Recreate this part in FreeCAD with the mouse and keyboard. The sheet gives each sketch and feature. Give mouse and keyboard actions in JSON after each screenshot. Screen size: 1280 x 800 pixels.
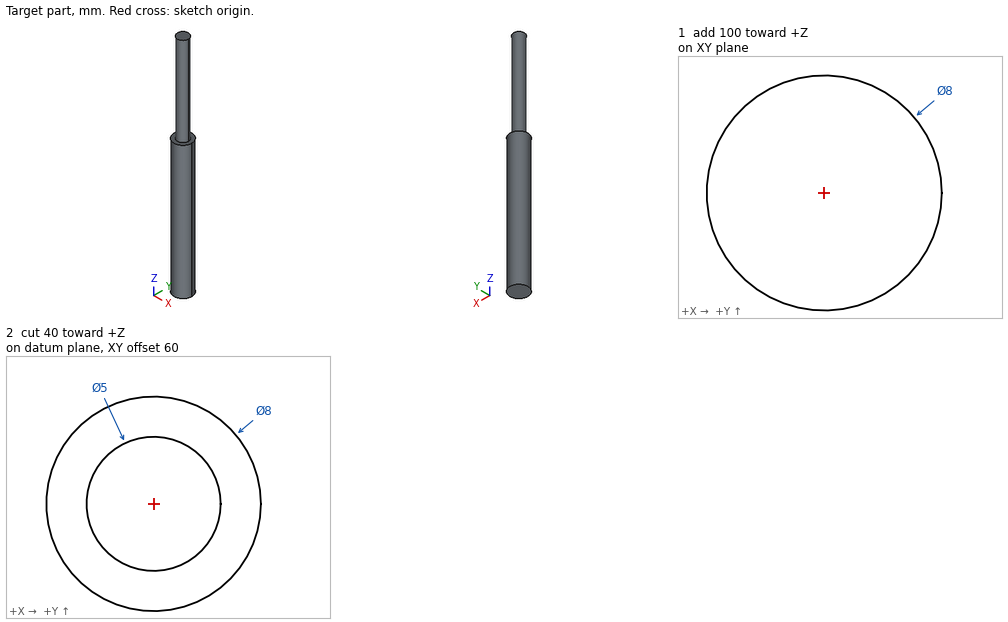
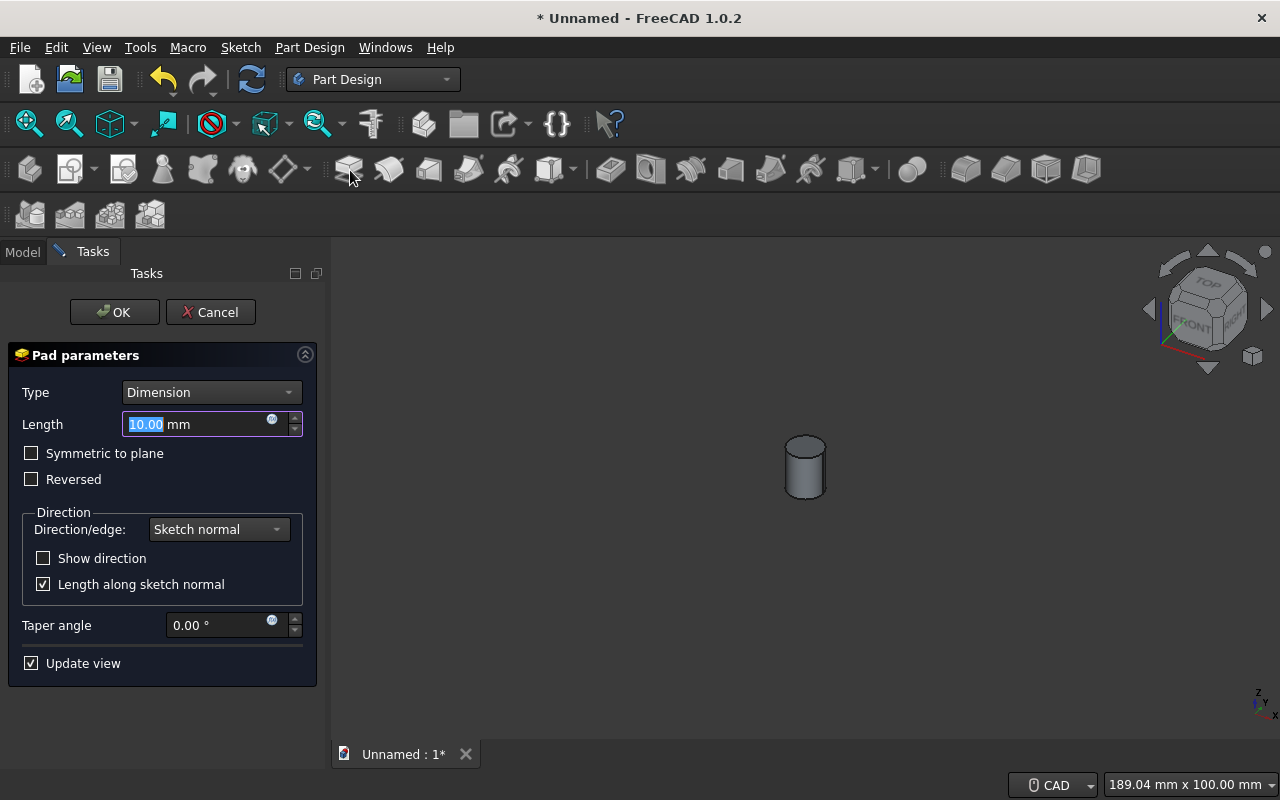
{"action": "type", "text": "100"}
{"action": "key", "text": "Tab"}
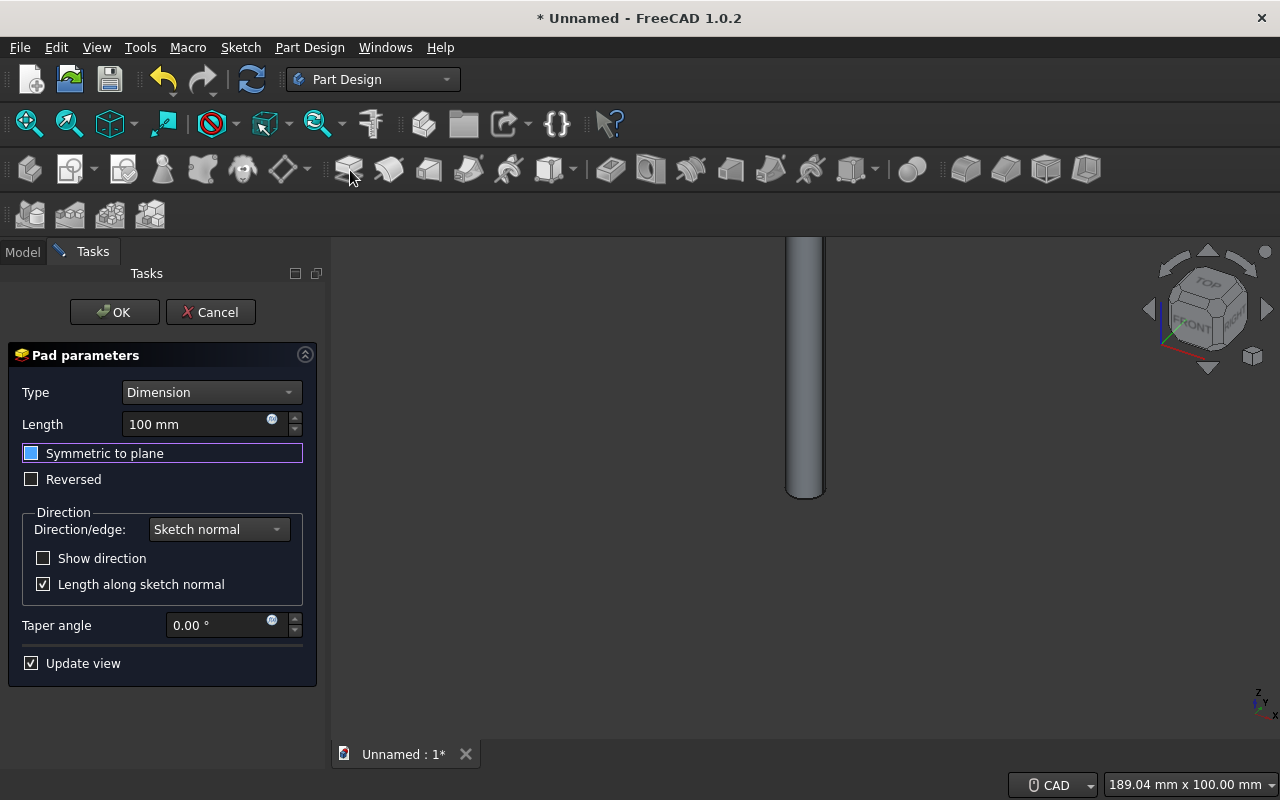
{"action": "left_click", "coordinate": [115, 312]}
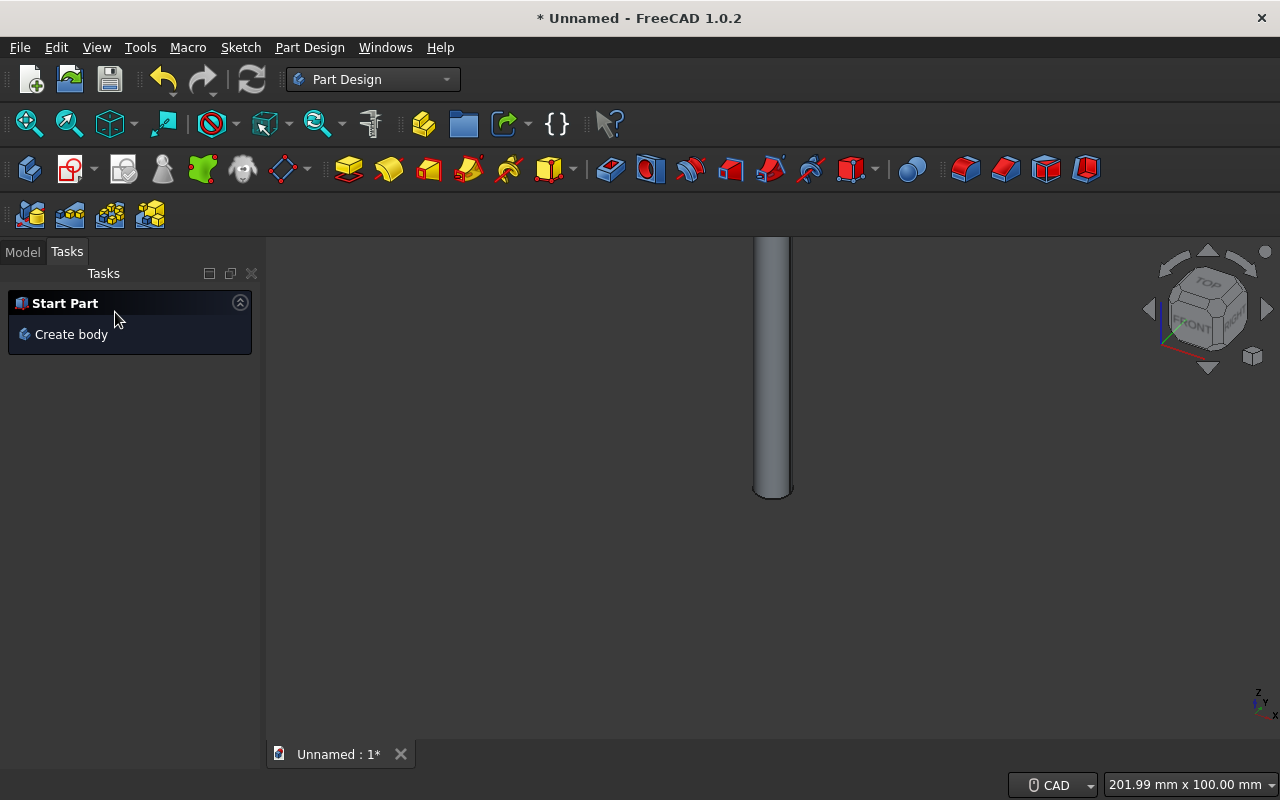
{"action": "left_click", "coordinate": [30, 124]}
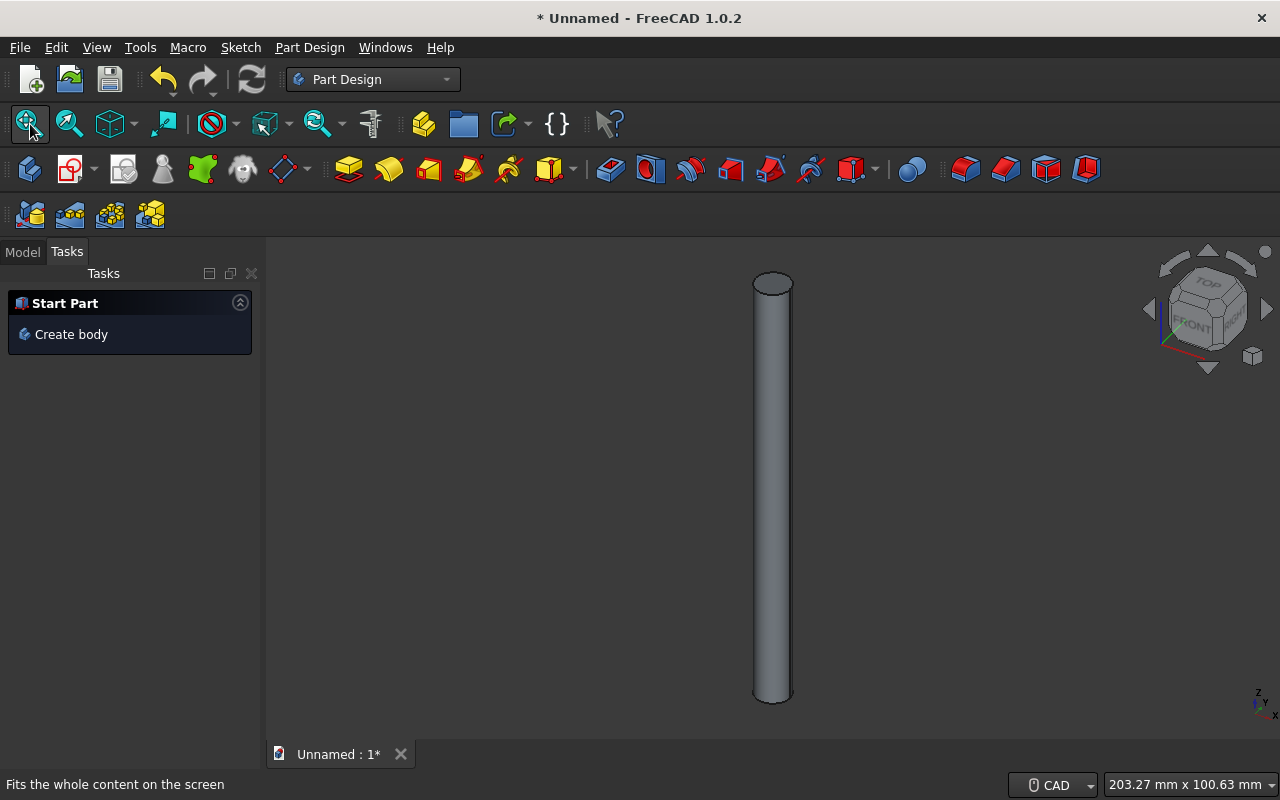
{"action": "left_click", "coordinate": [23, 251]}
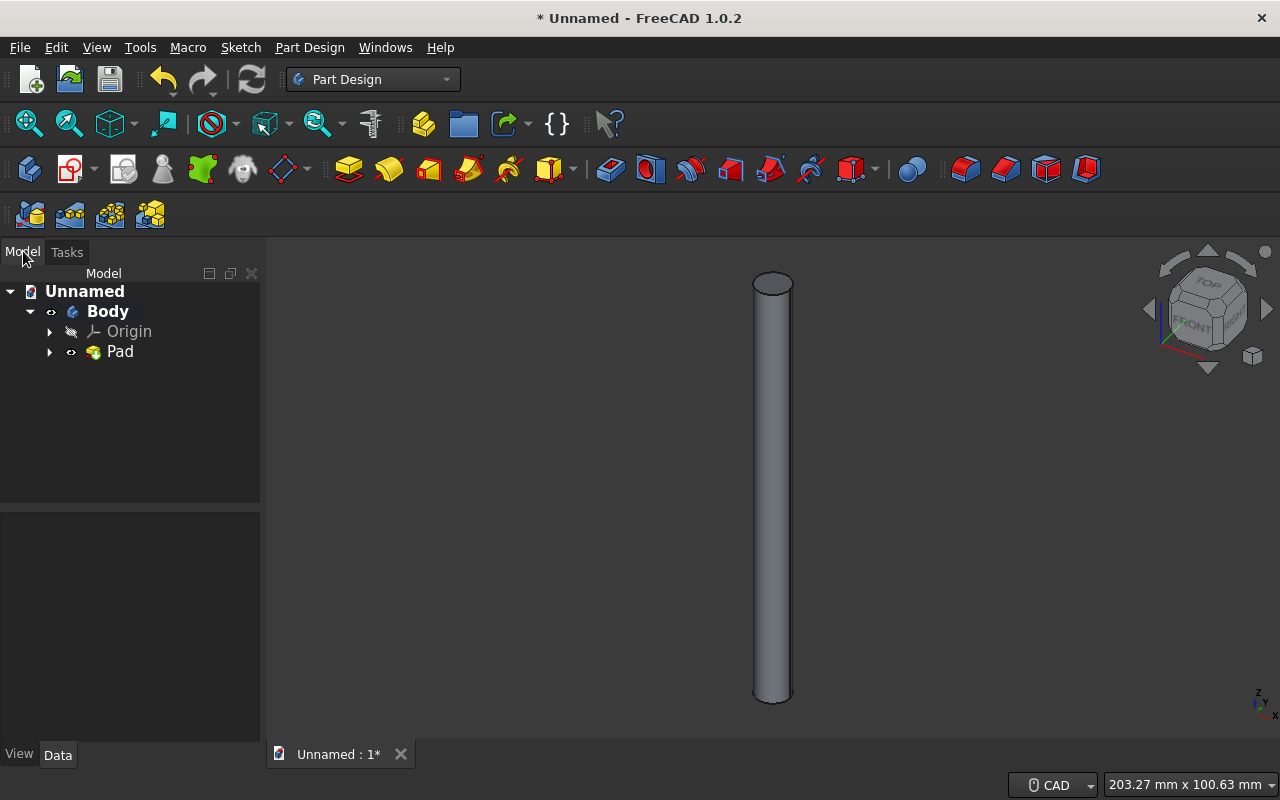
{"action": "left_click", "coordinate": [50, 332]}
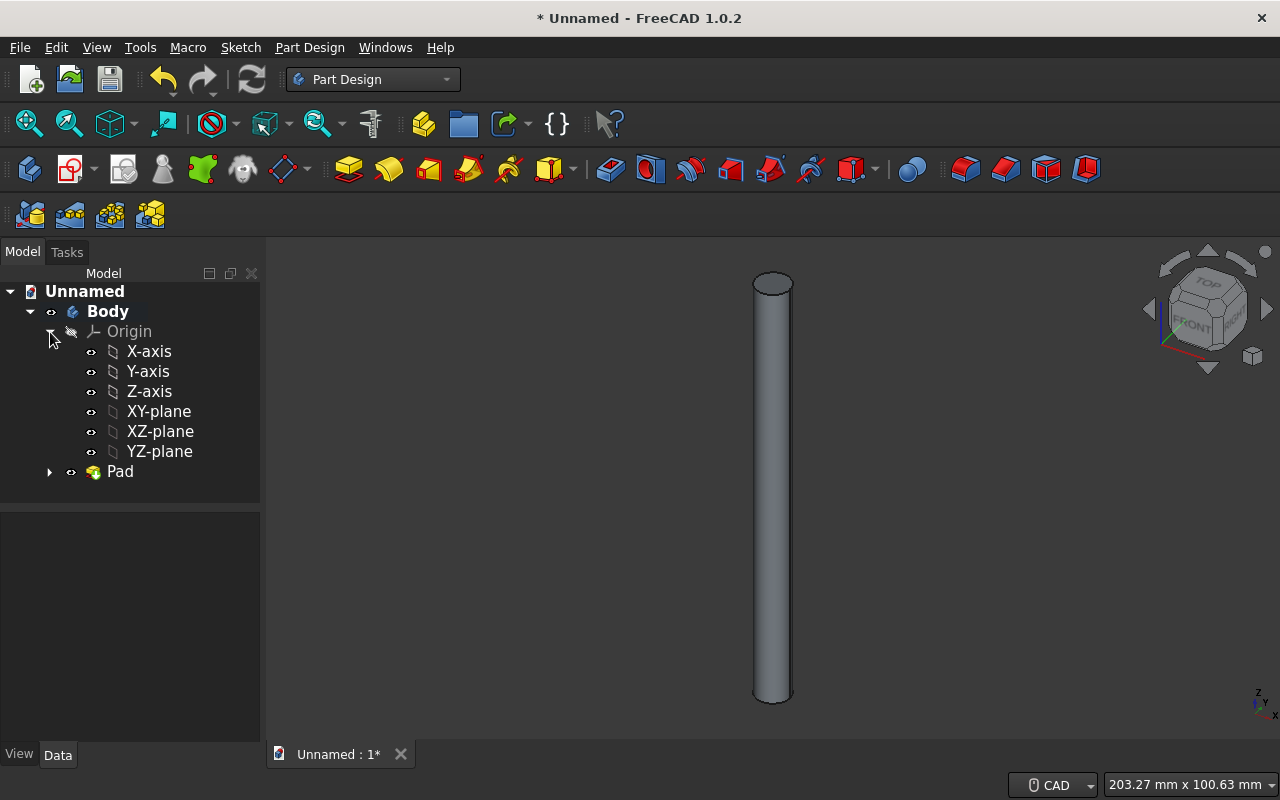
{"action": "left_click", "coordinate": [136, 412]}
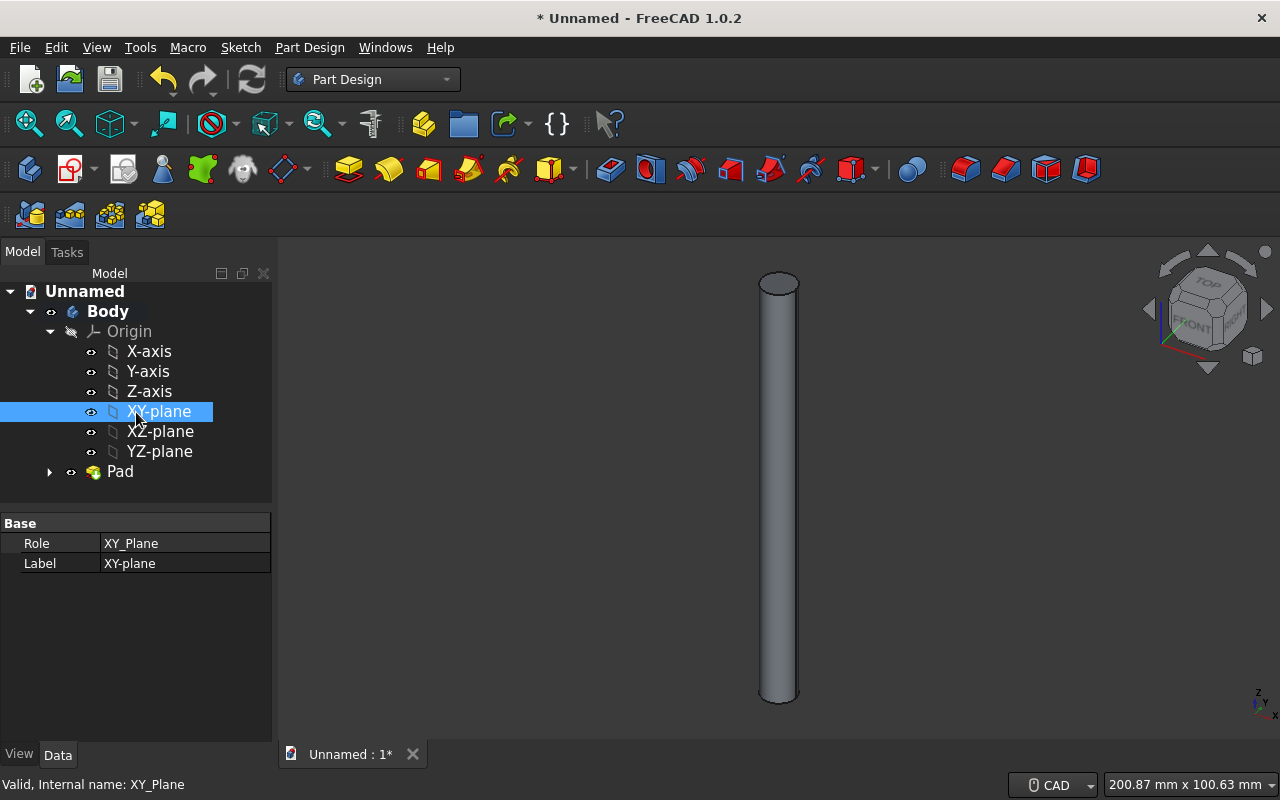
{"action": "left_click", "coordinate": [284, 170]}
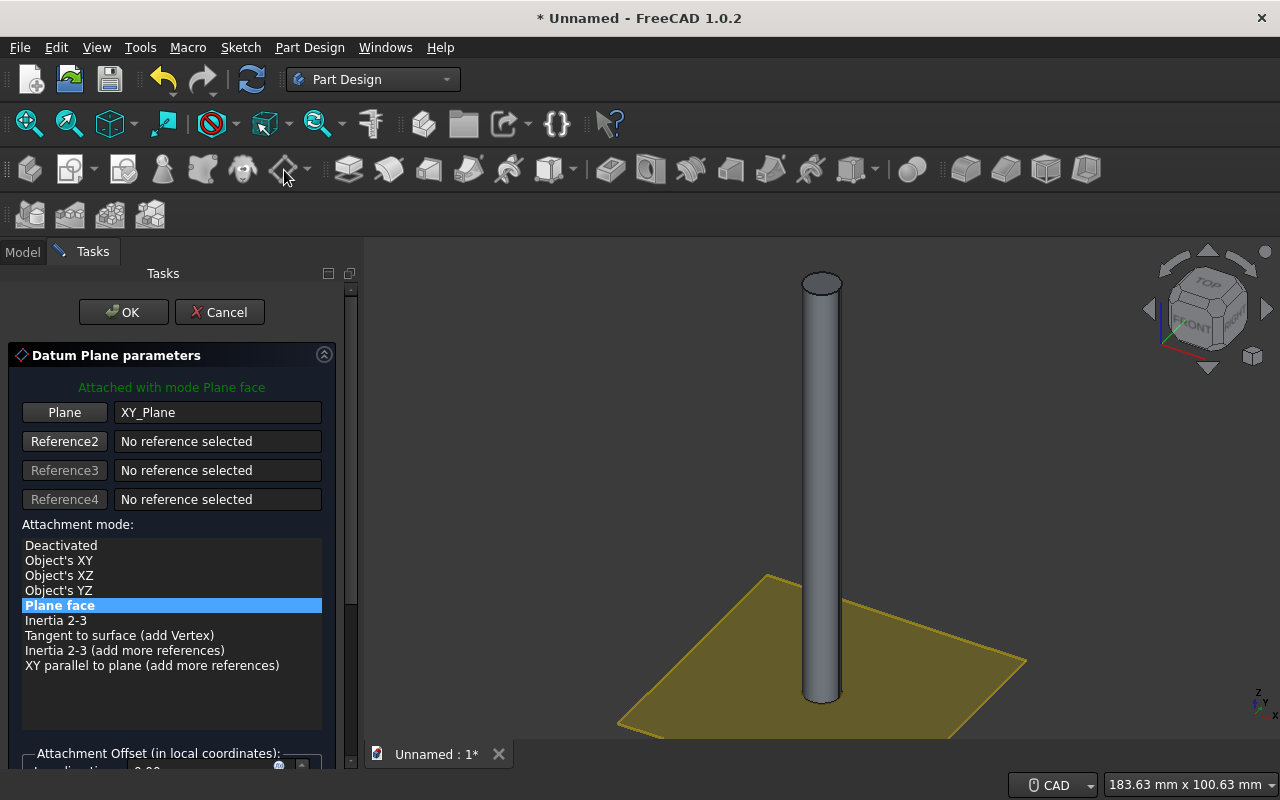
{"action": "scroll", "coordinate": [351, 526], "scroll_direction": "down", "scroll_amount": 3}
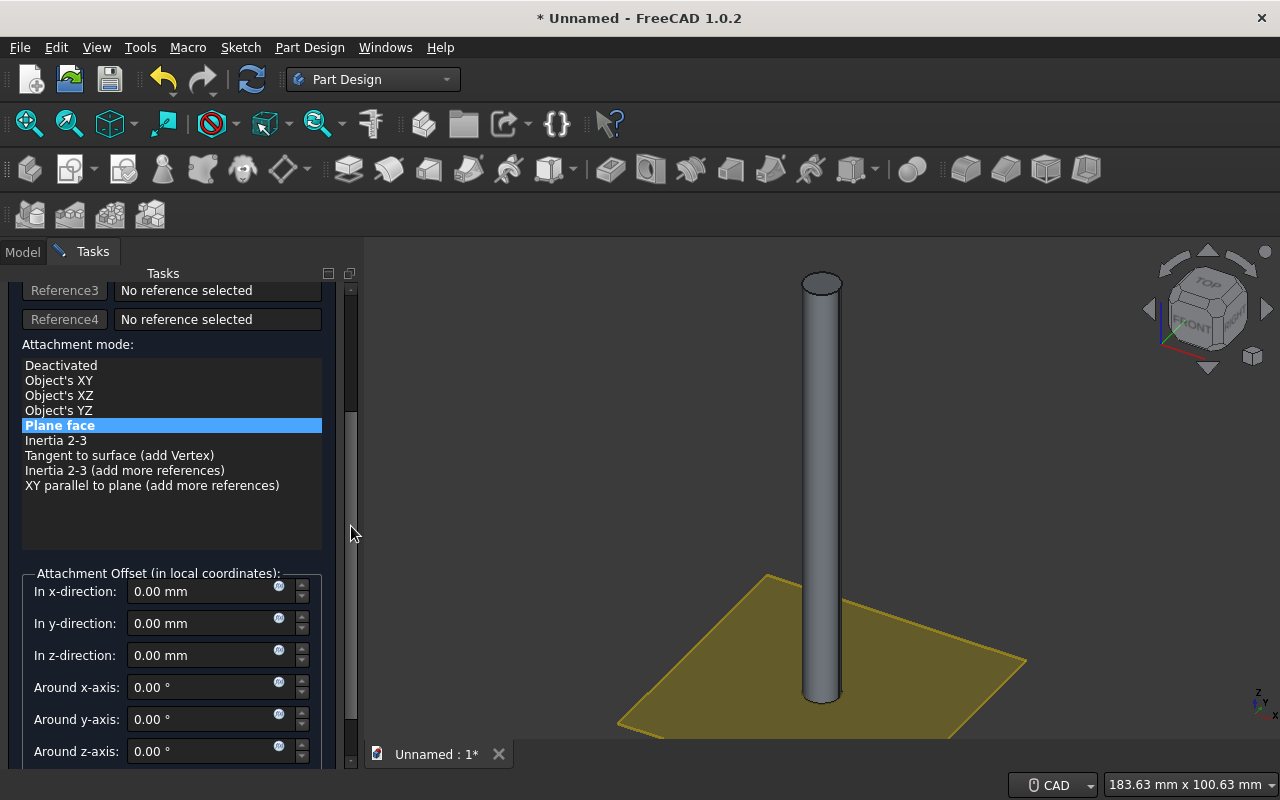
{"action": "triple_click", "coordinate": [210, 655]}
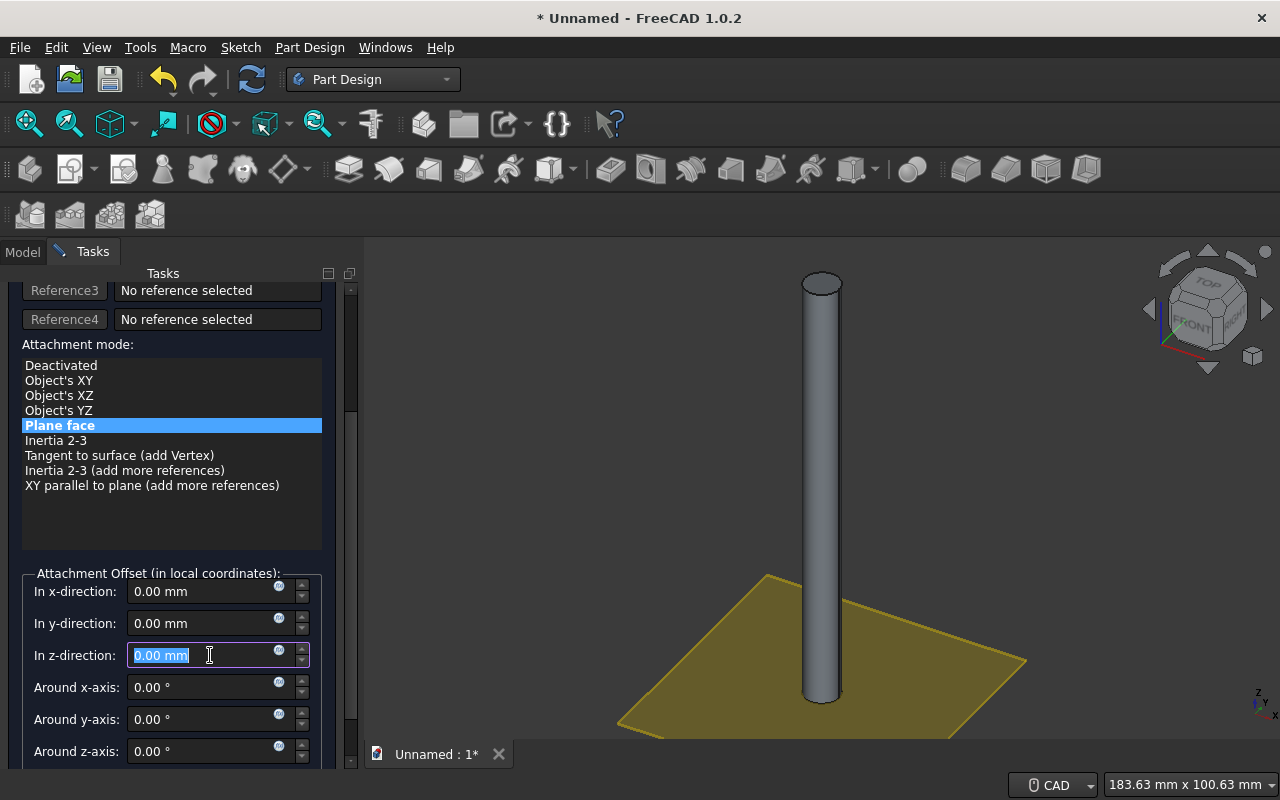
{"action": "type", "text": "60"}
{"action": "key", "text": "Tab"}